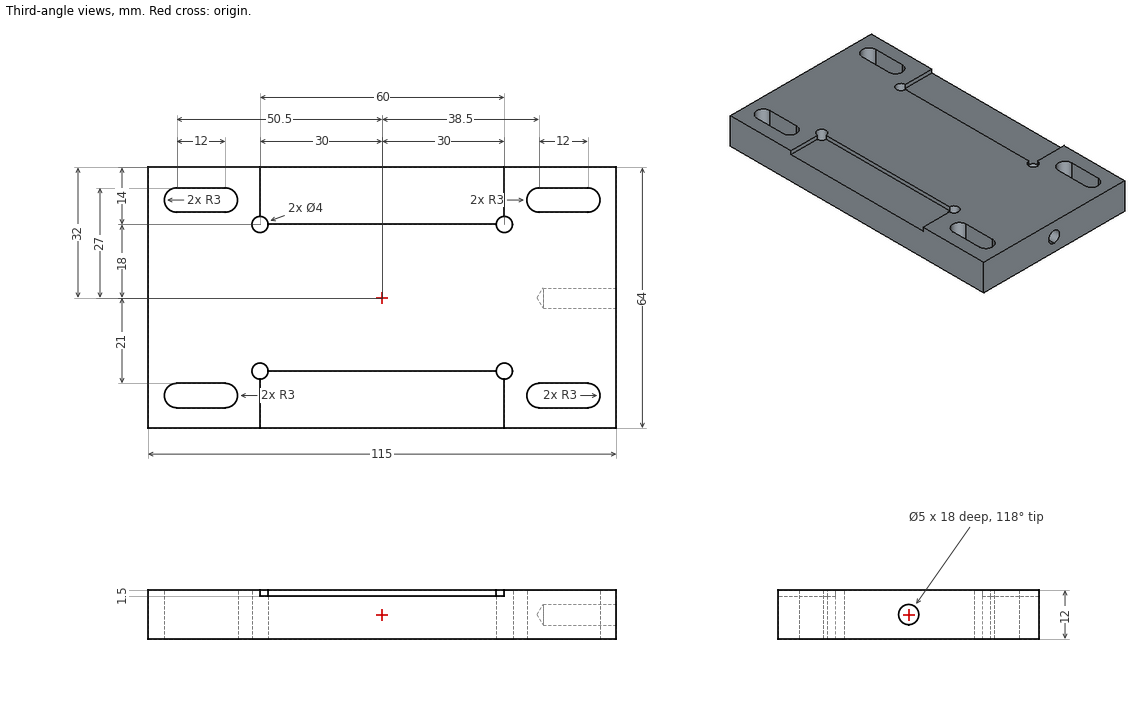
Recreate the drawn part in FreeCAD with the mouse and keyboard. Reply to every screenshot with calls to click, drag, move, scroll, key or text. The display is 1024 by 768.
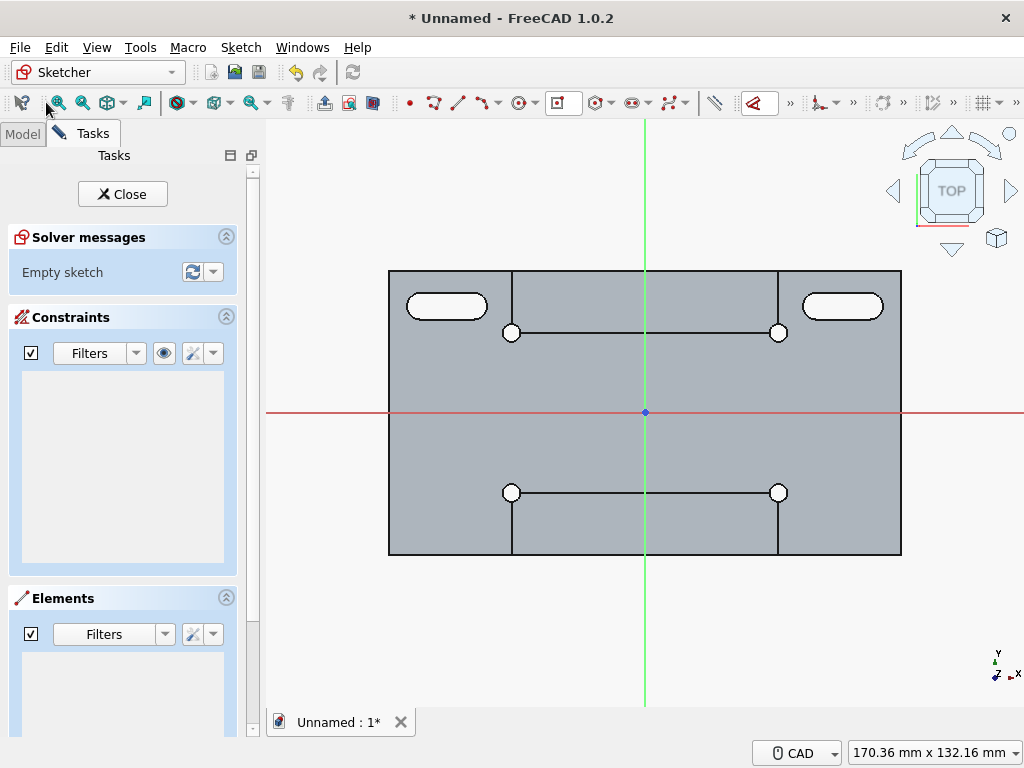
scroll(414, 547, up, 8)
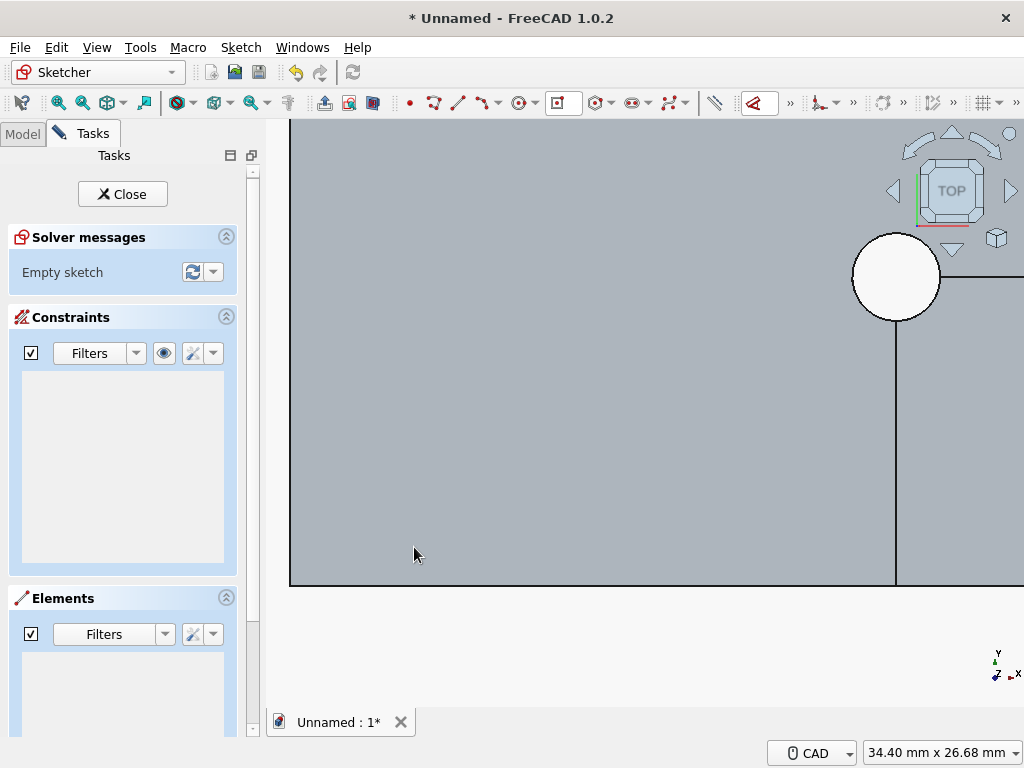
key(g)
key(s)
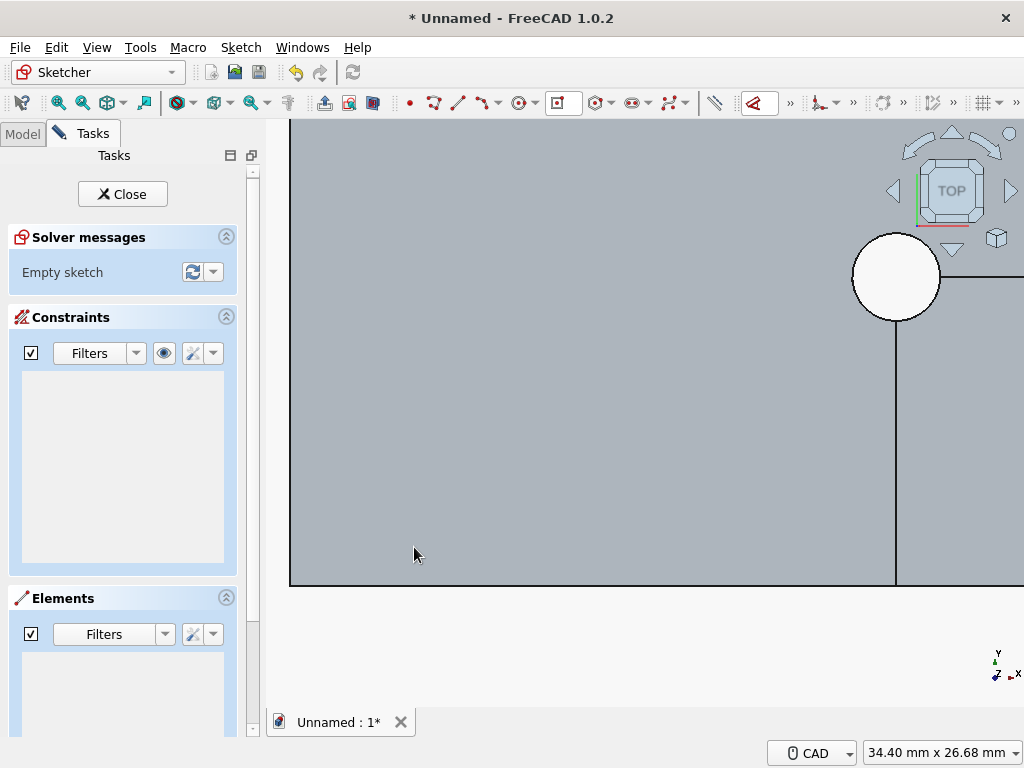
click(444, 409)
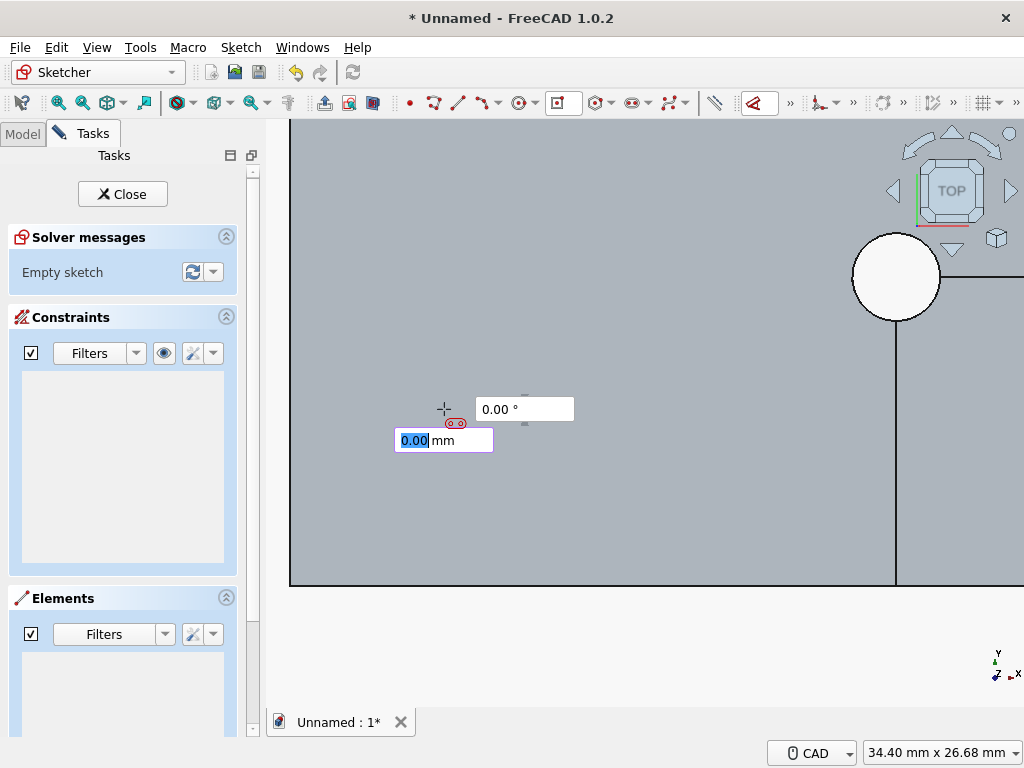
click(709, 409)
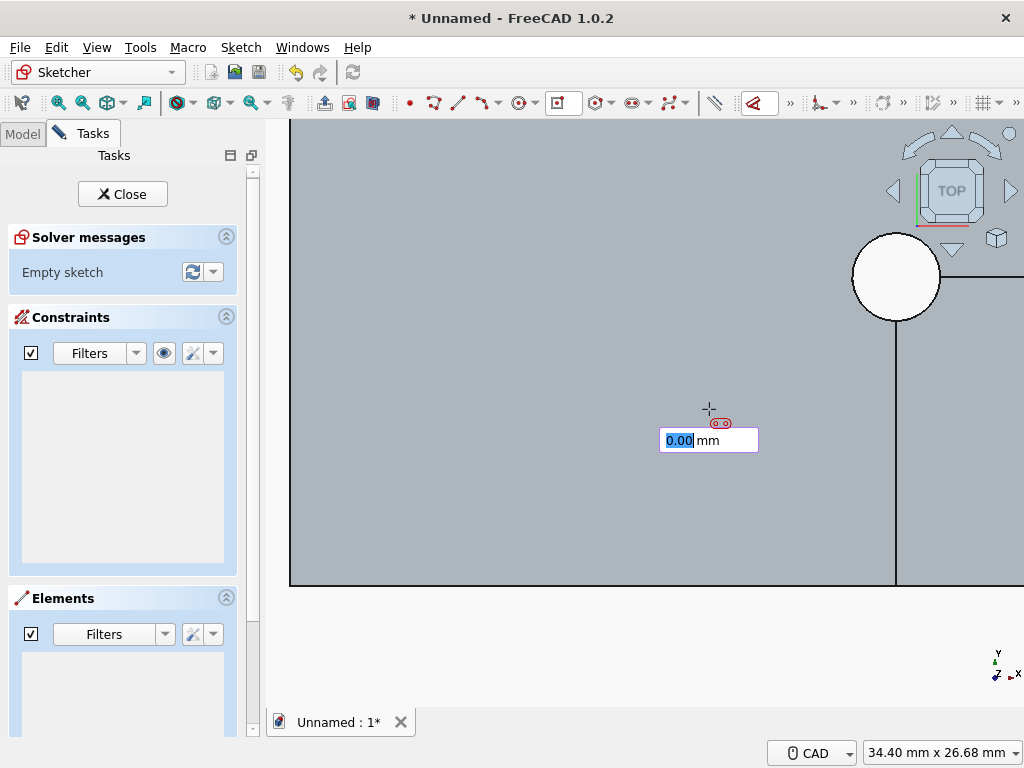
click(577, 475)
key(Escape)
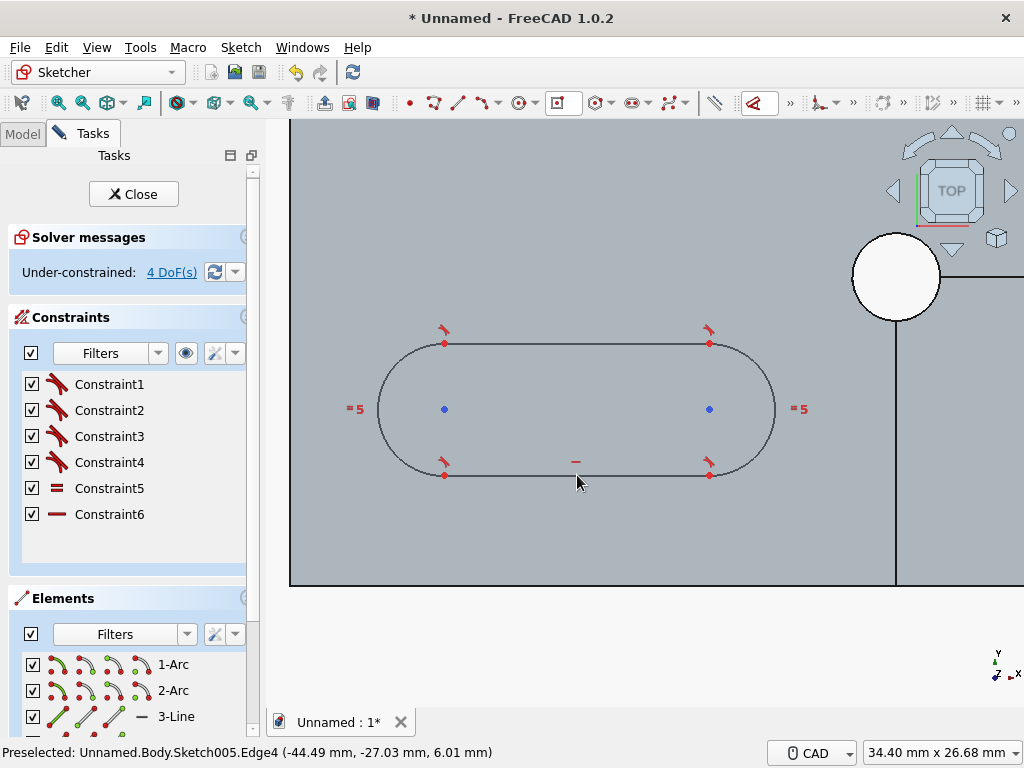
click(391, 371)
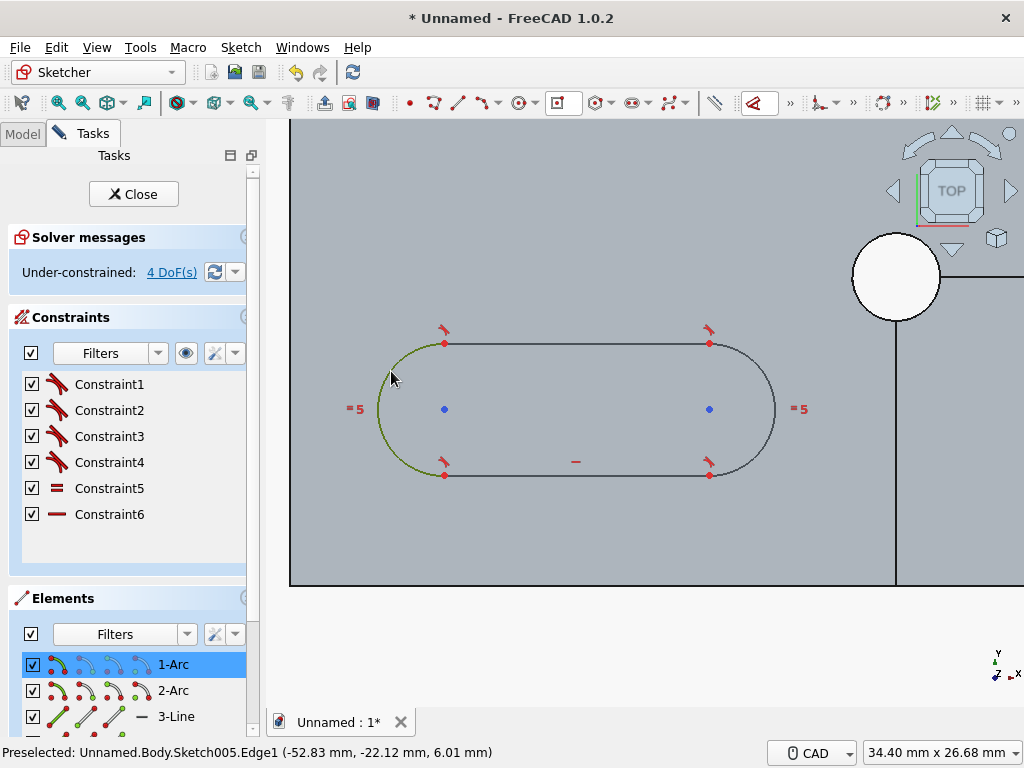
key(k)
key(r)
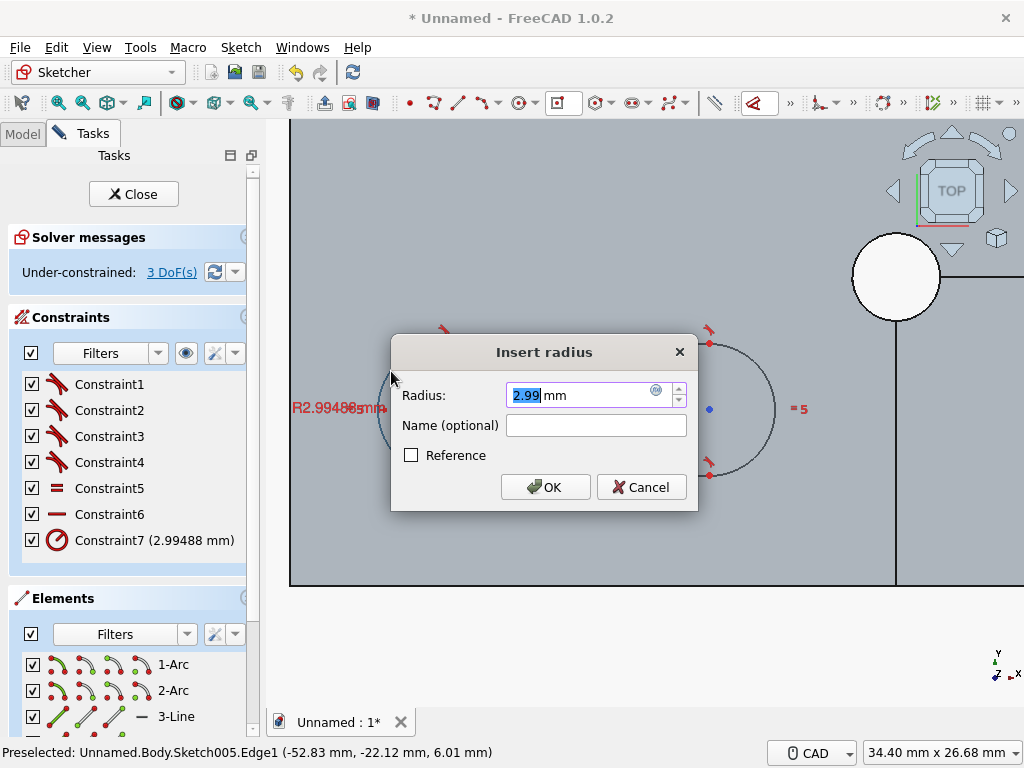
text(3)
key(Return)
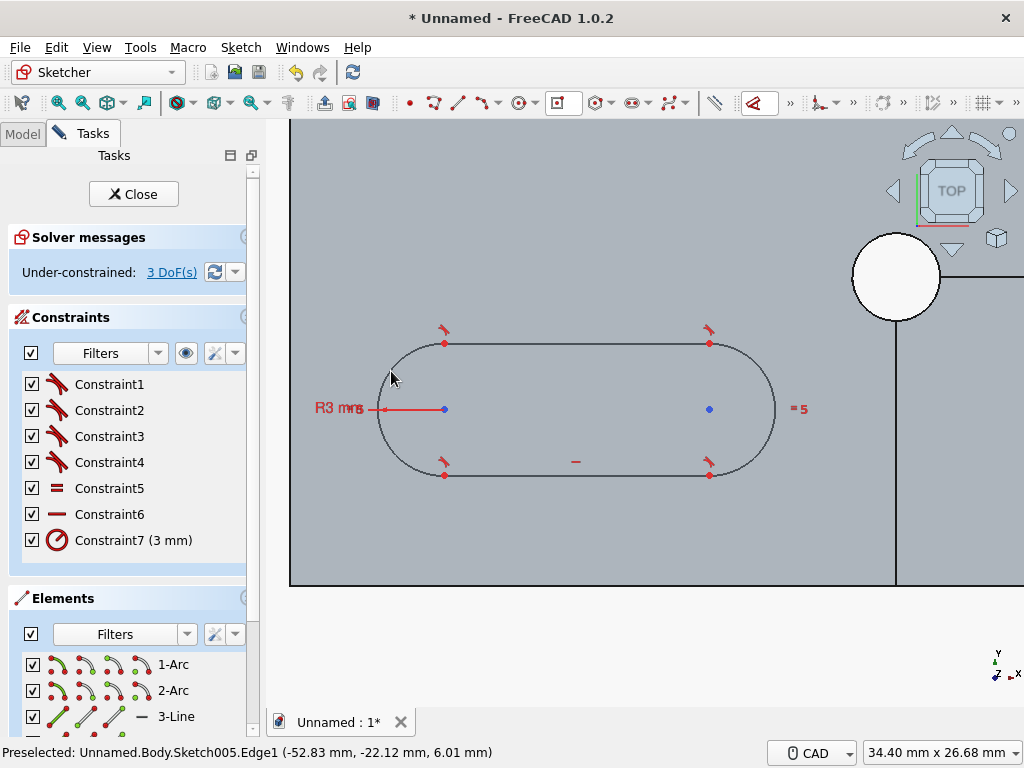
click(524, 344)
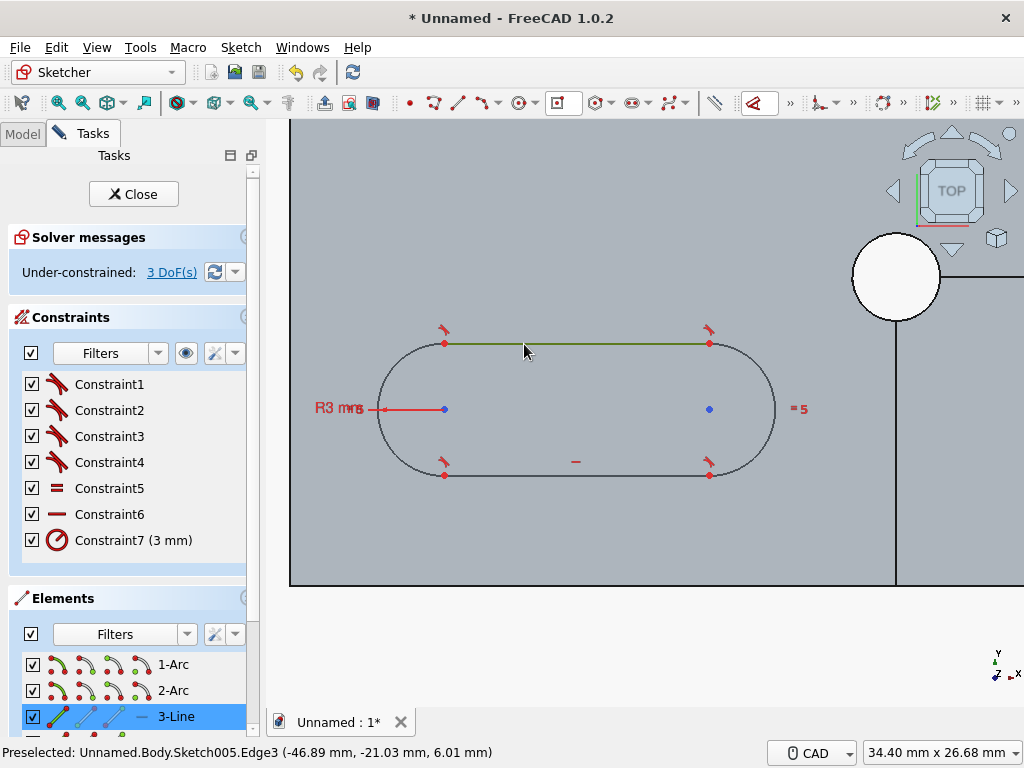
key(l)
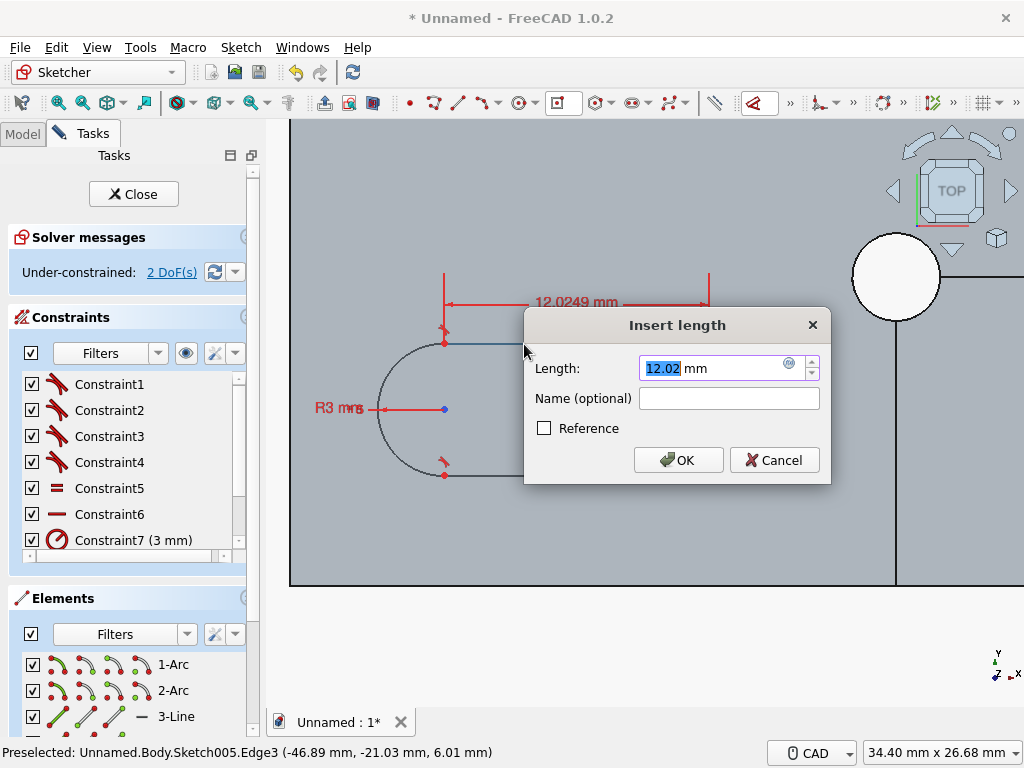
text(12)
key(Return)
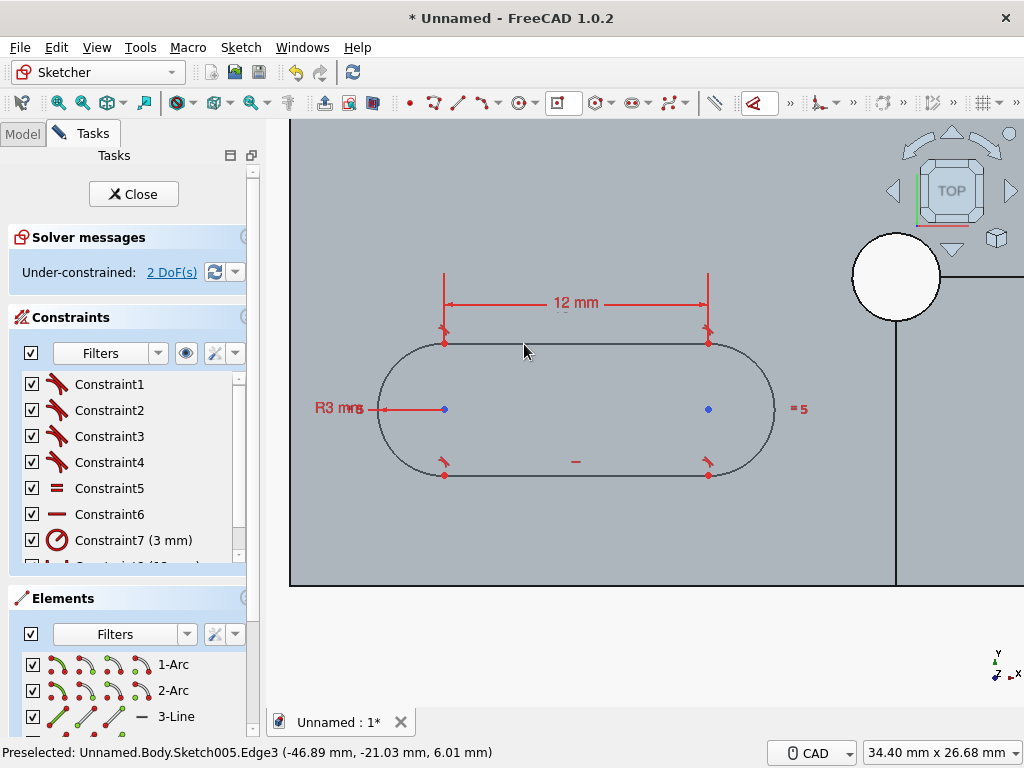
click(444, 344)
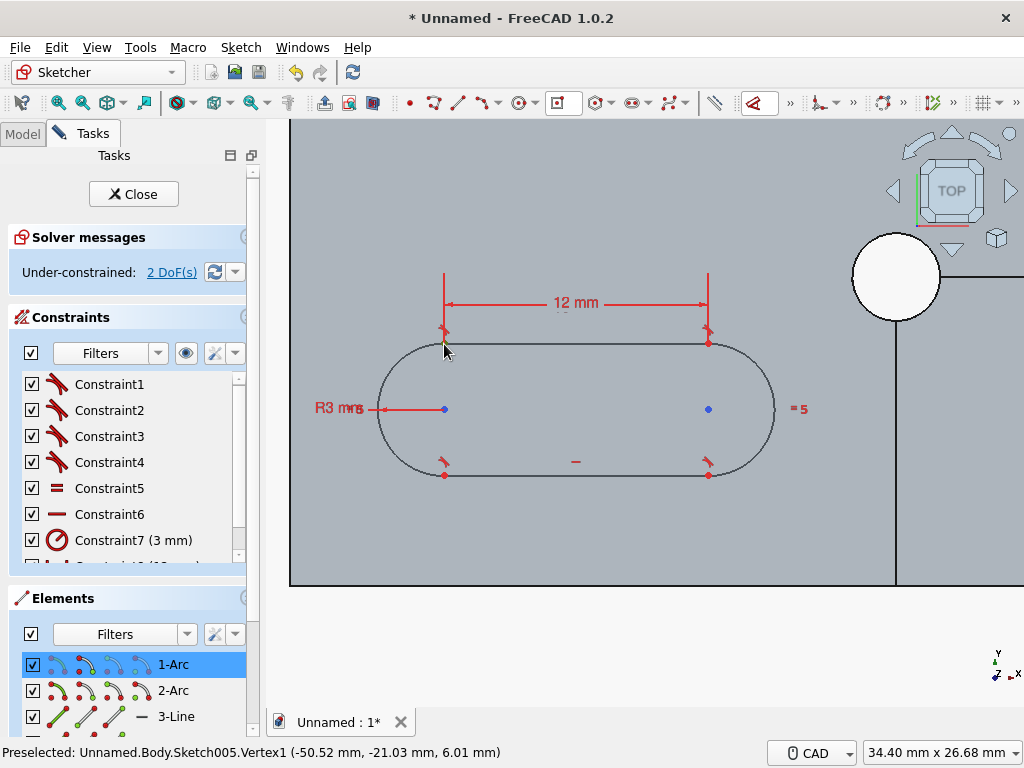
key(i)